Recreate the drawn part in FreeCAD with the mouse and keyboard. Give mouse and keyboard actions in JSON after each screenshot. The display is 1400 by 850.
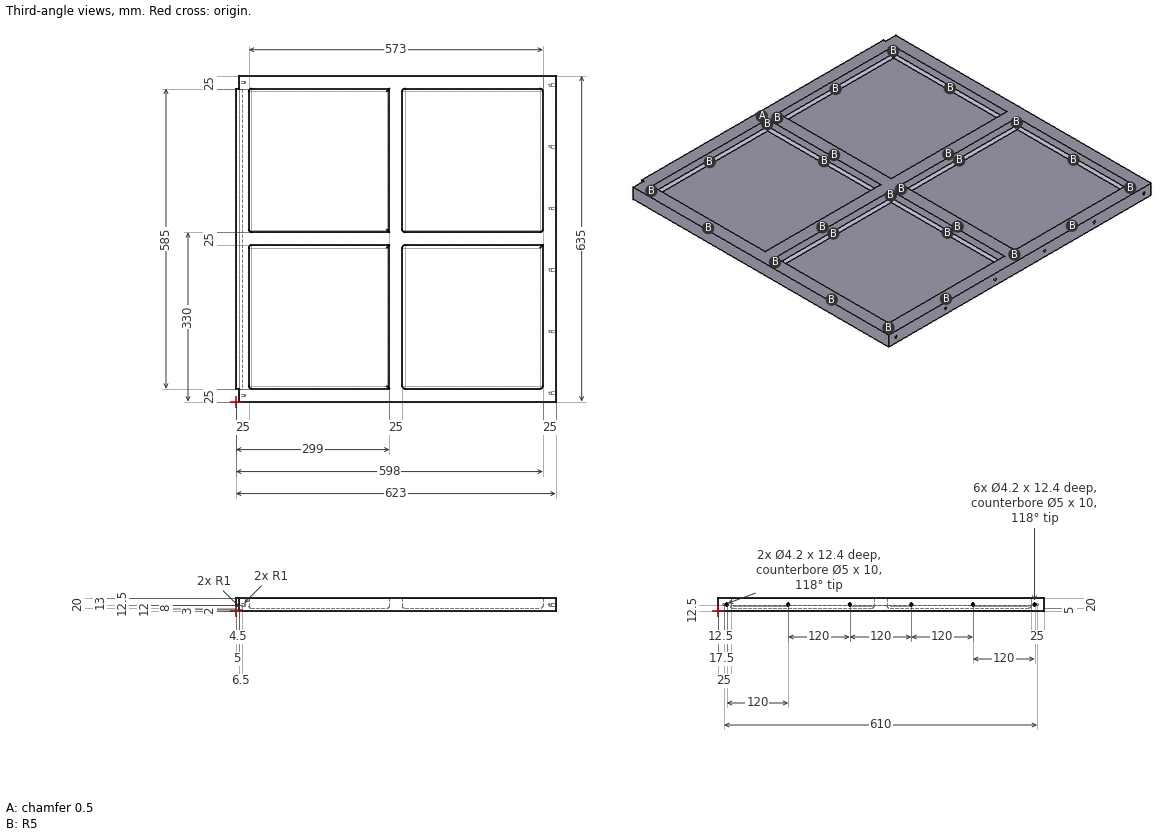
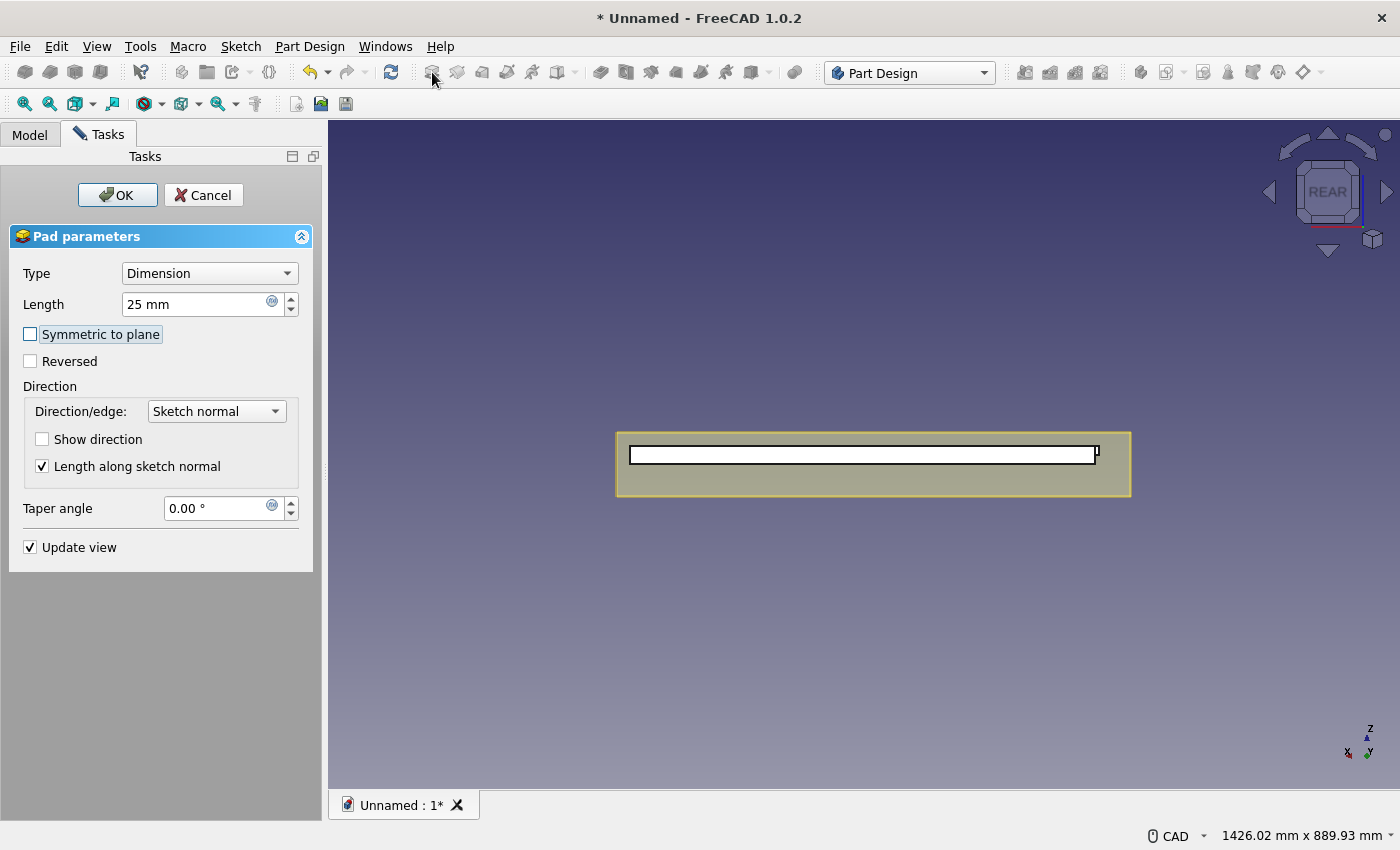
{"action": "left_click", "coordinate": [118, 195]}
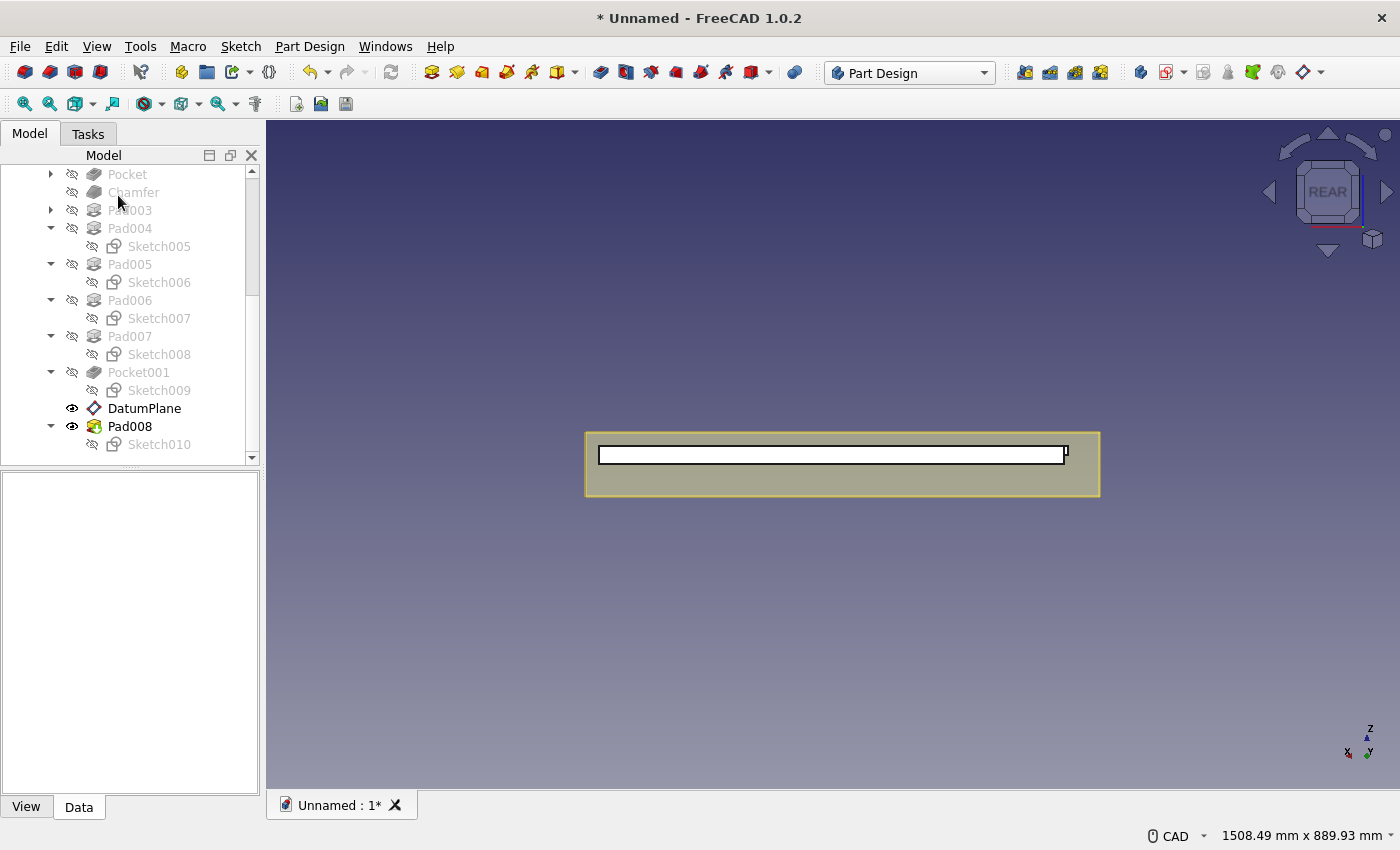
{"action": "left_click", "coordinate": [117, 408]}
{"action": "key", "text": "space"}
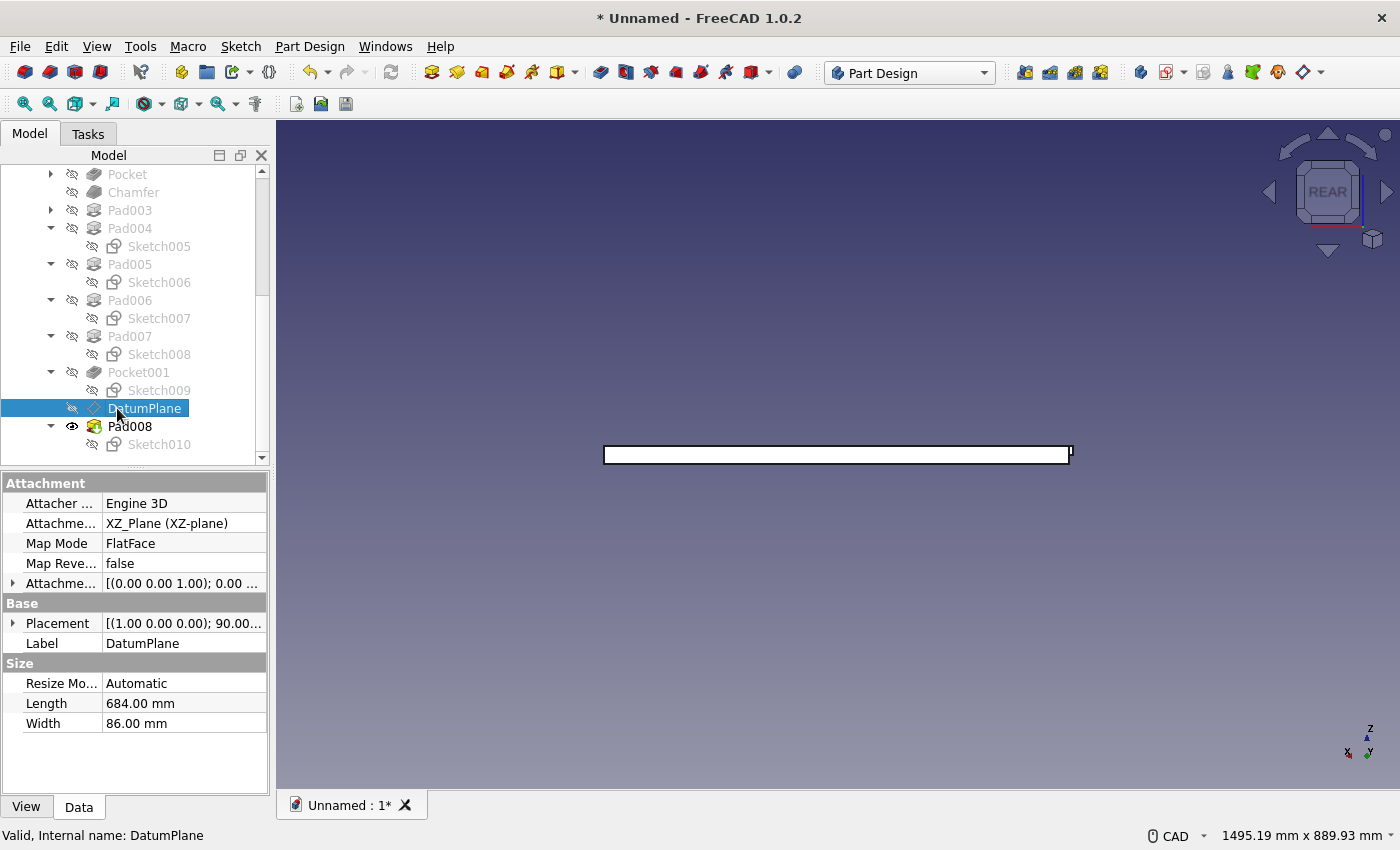
{"action": "left_click", "coordinate": [25, 104]}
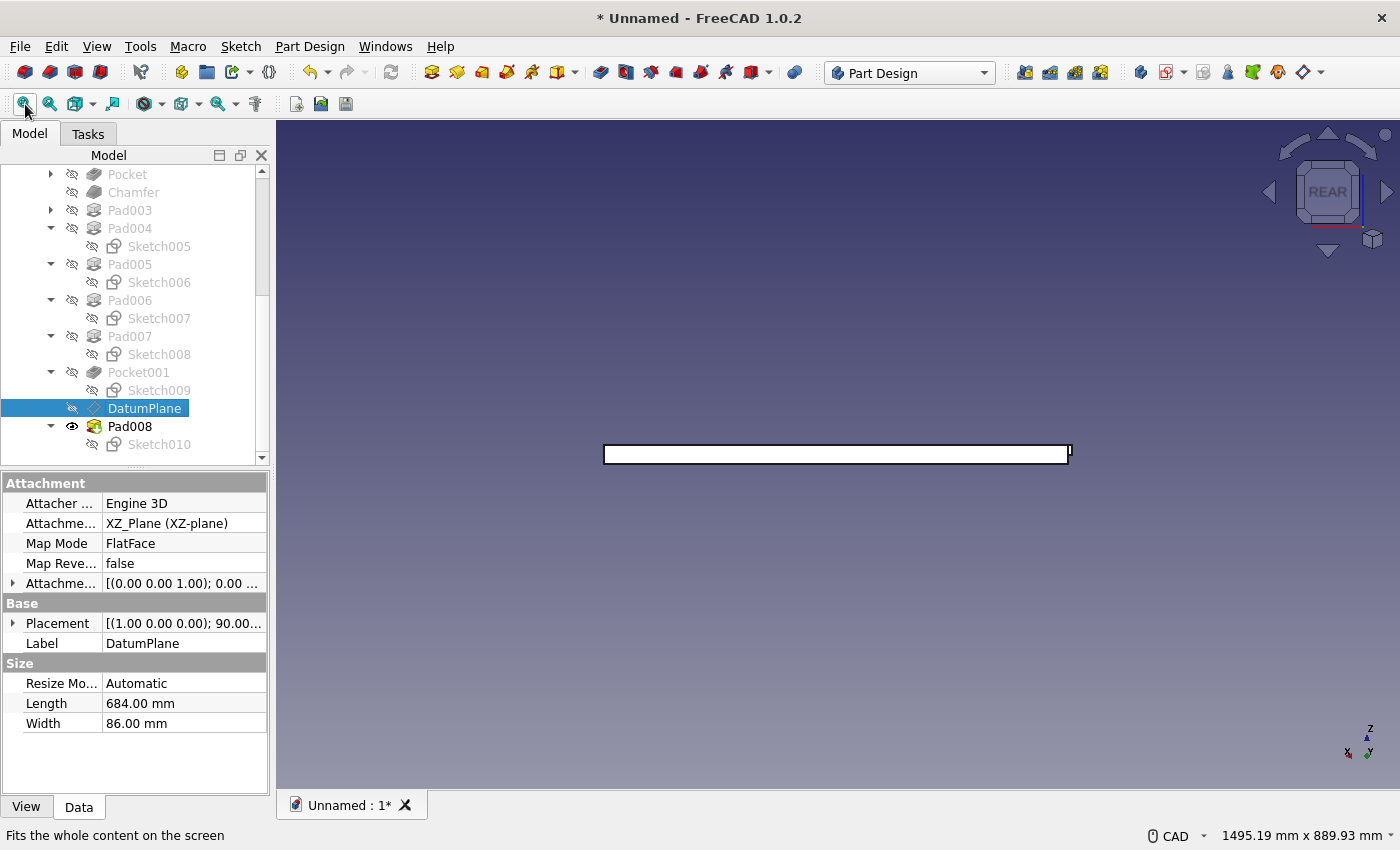
{"action": "left_click", "coordinate": [316, 749]}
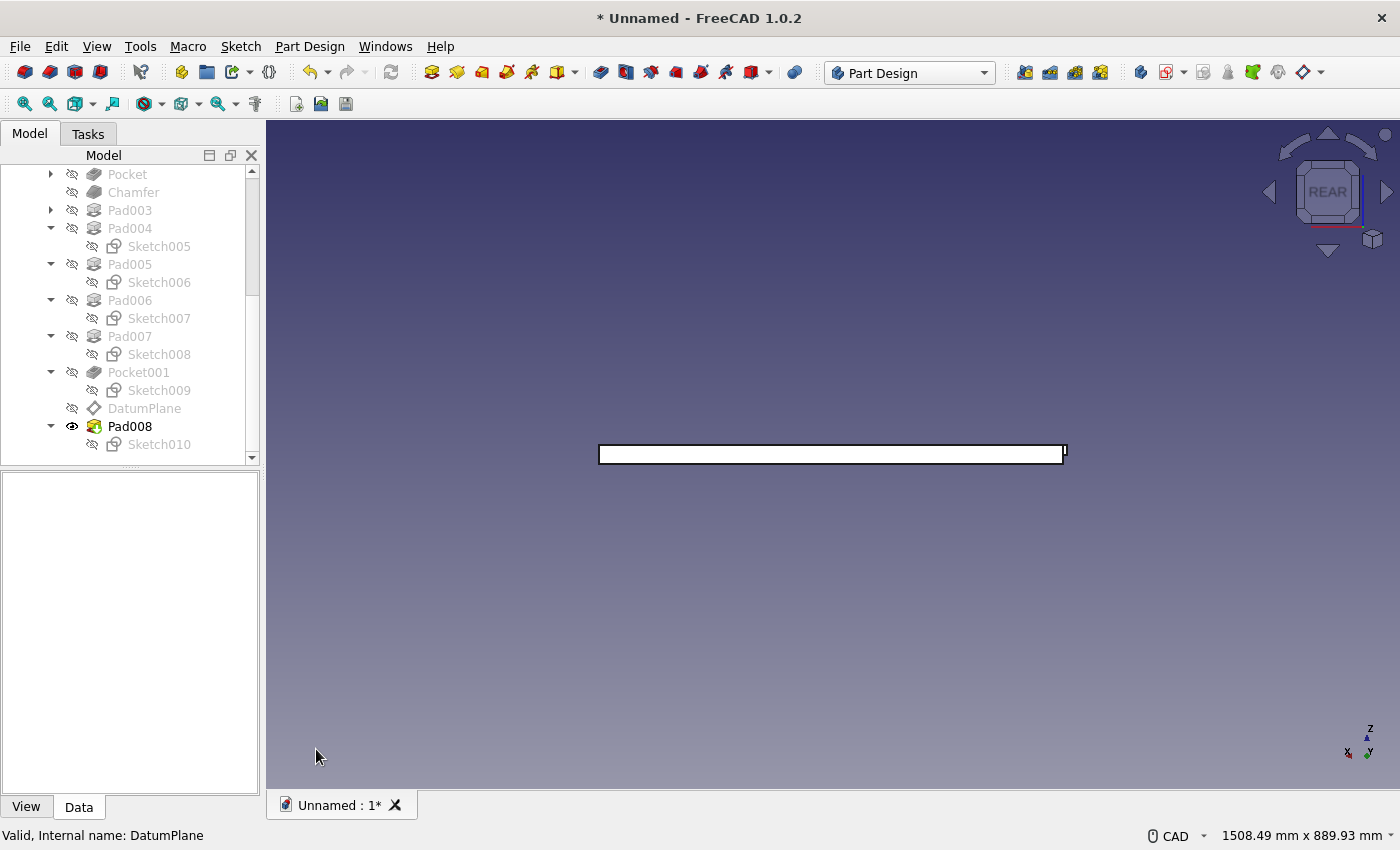
{"action": "left_click", "coordinate": [1166, 72]}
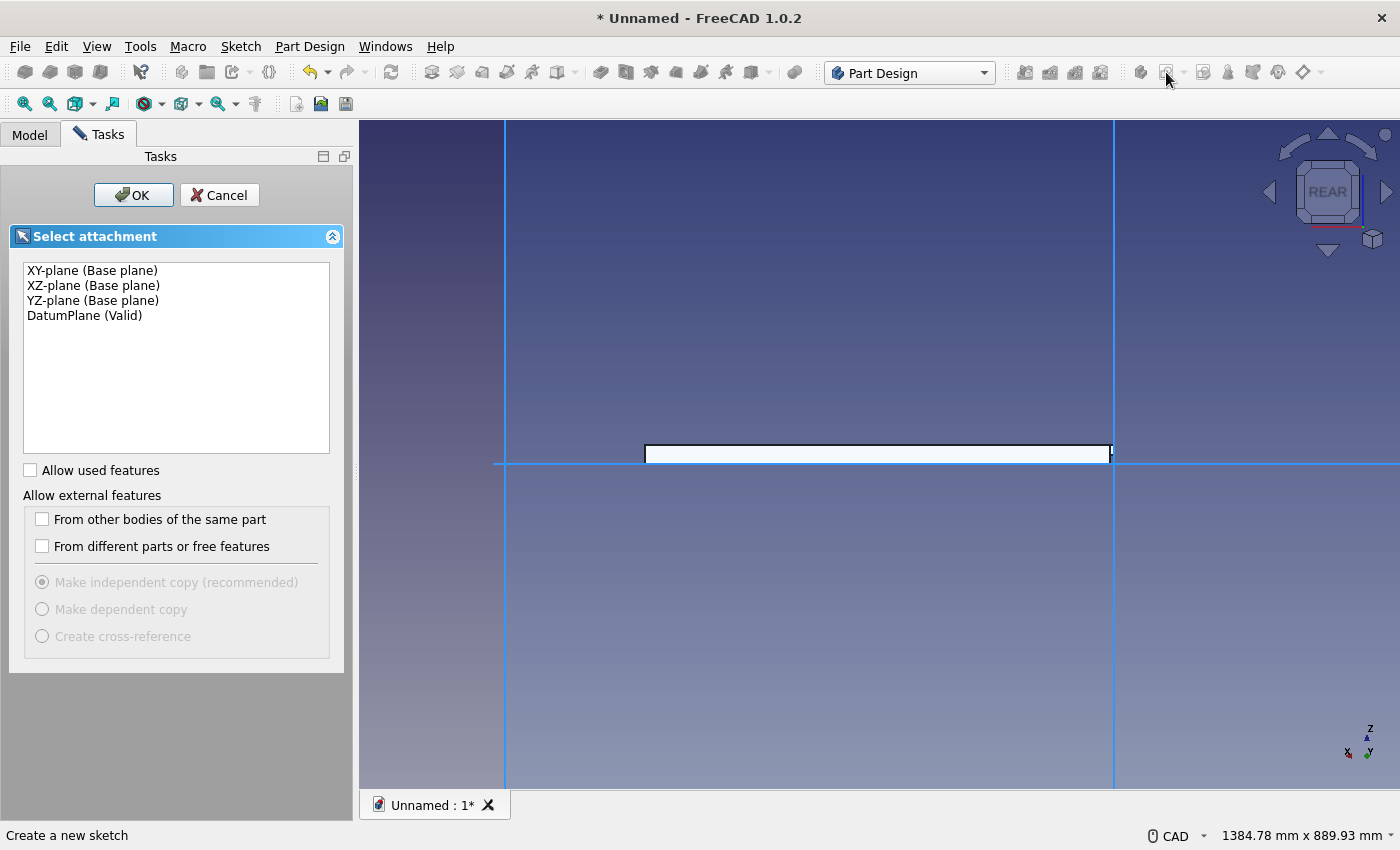
{"action": "left_click", "coordinate": [84, 286]}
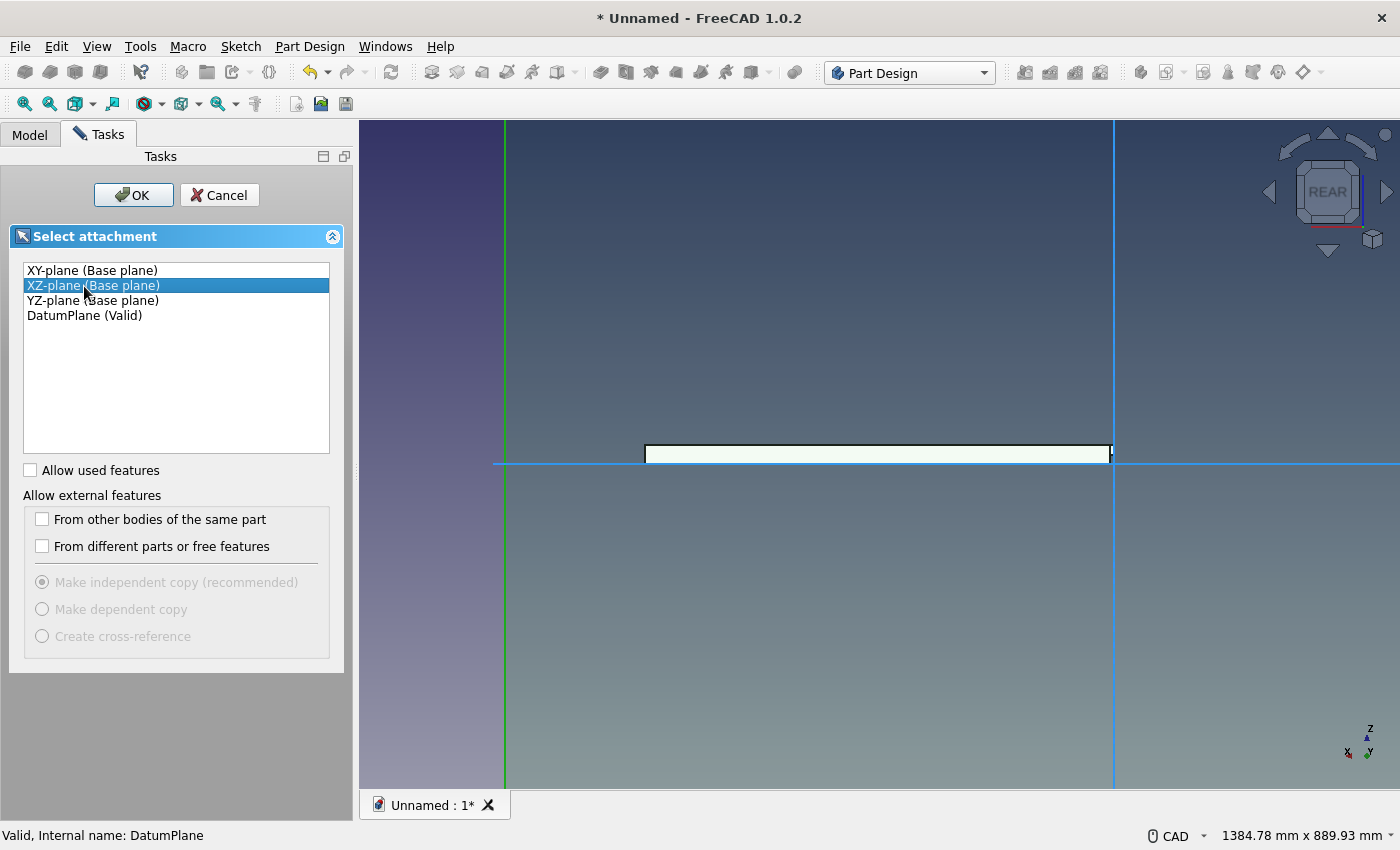
{"action": "left_click", "coordinate": [134, 195]}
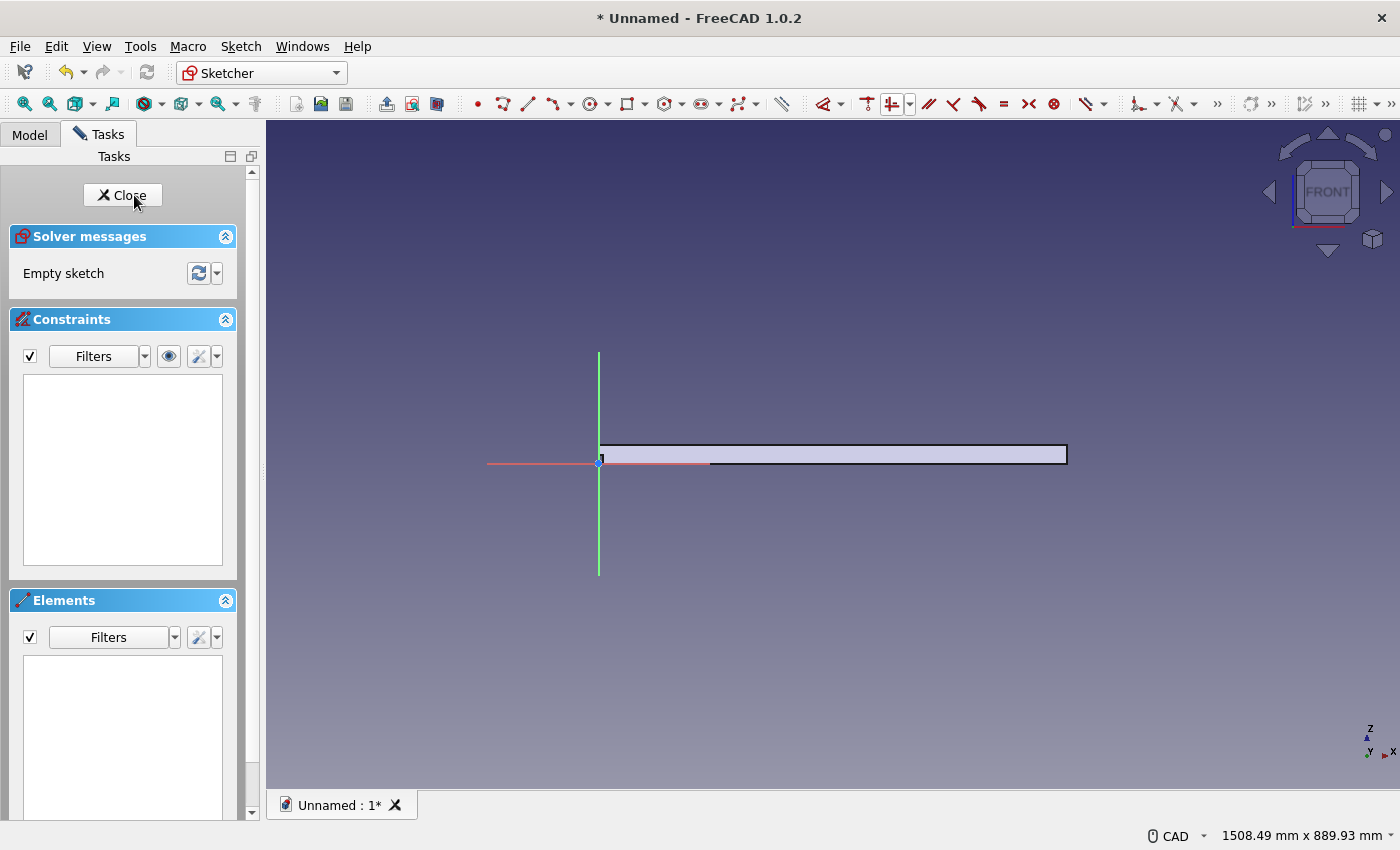
{"action": "scroll", "coordinate": [592, 455], "scroll_direction": "up", "scroll_amount": 15}